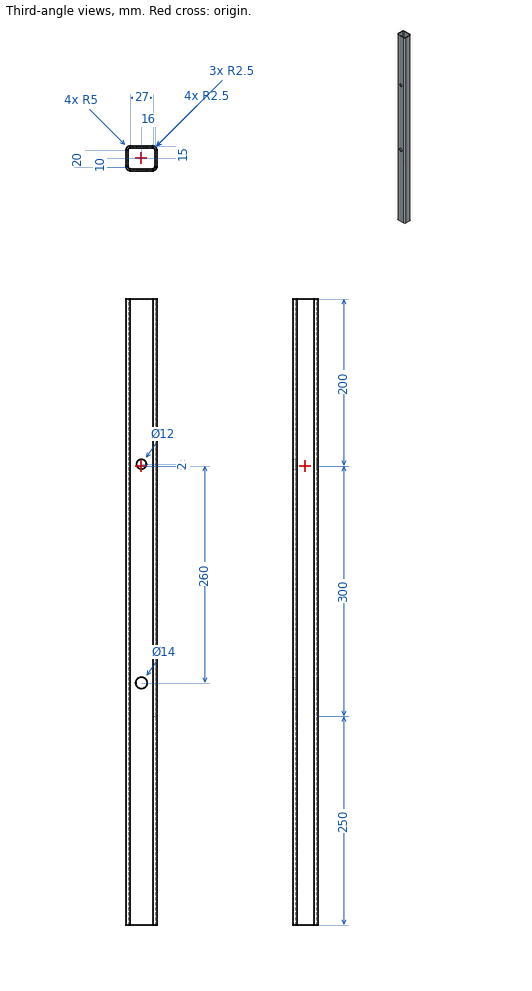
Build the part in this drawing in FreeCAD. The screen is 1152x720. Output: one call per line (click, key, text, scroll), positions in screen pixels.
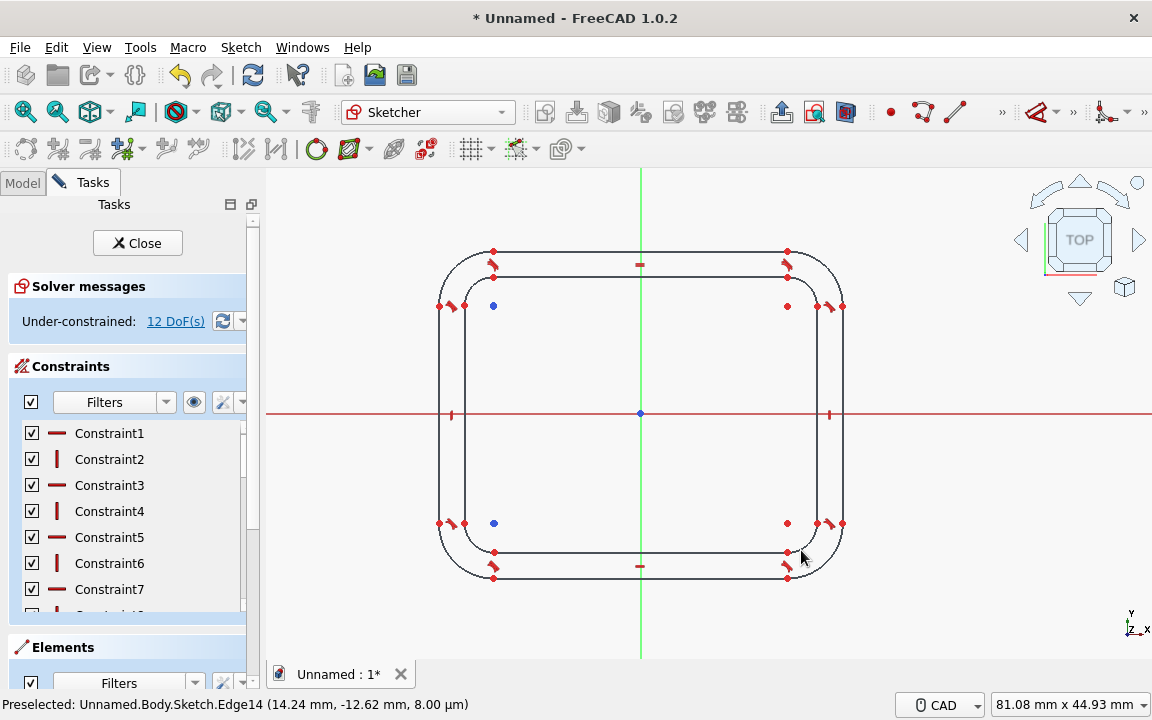
click(445, 549)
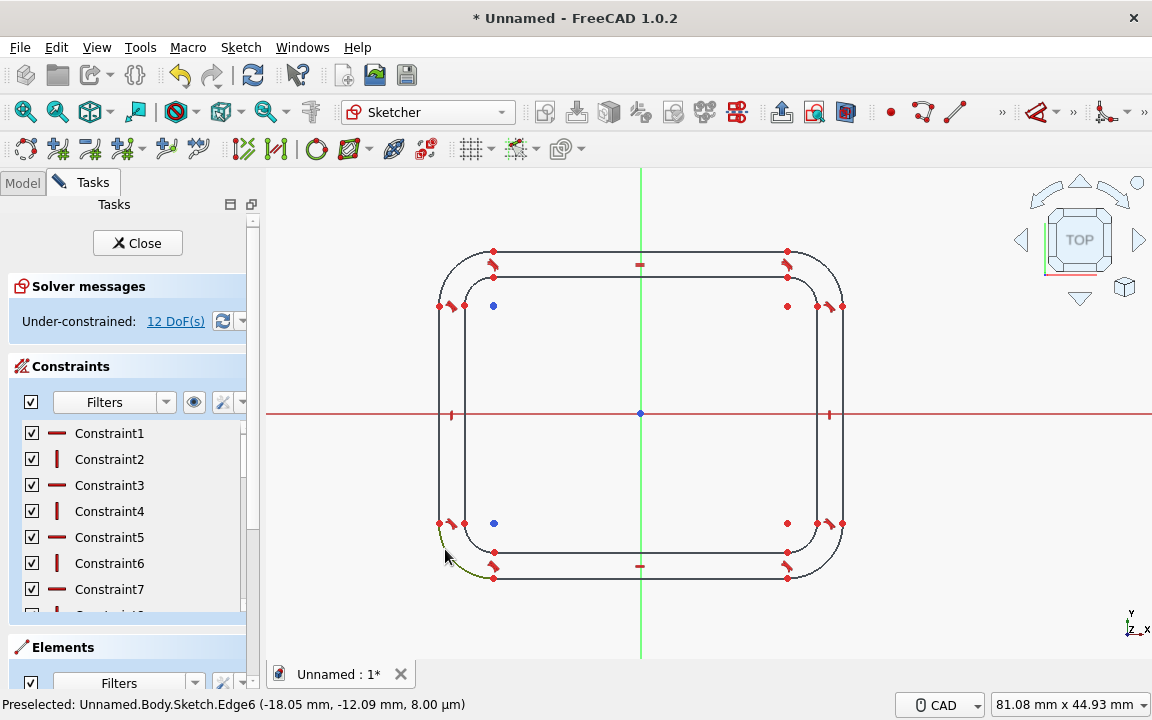
click(468, 537)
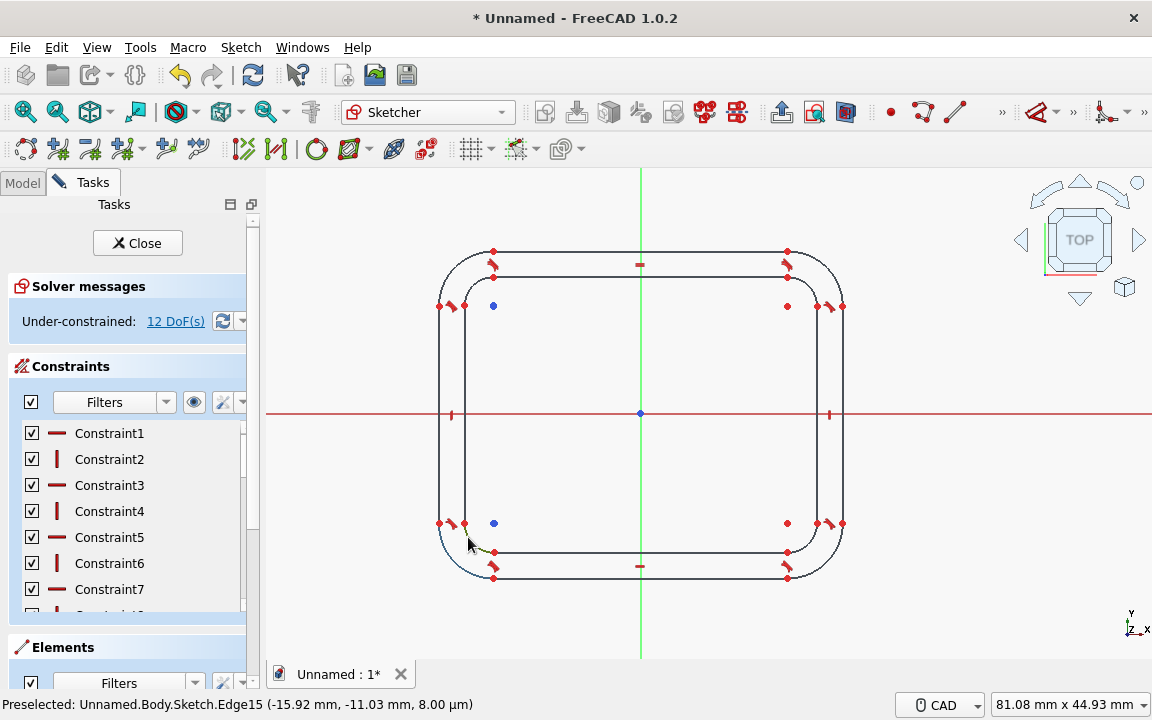
key(c)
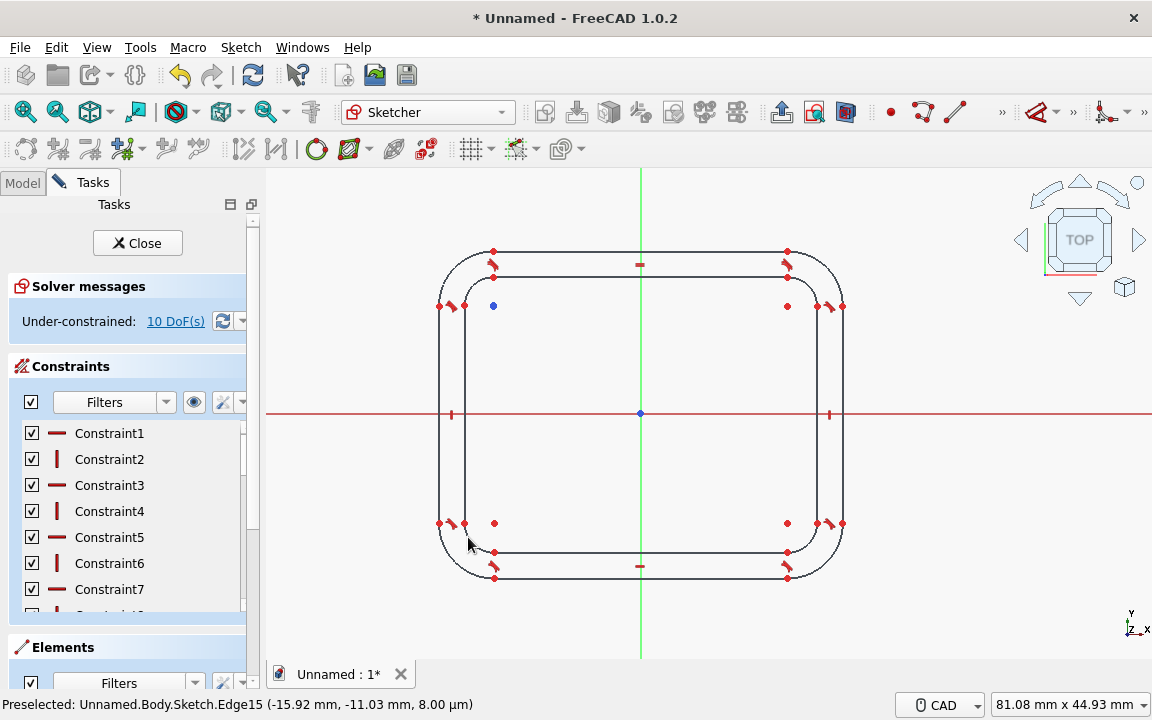
click(469, 257)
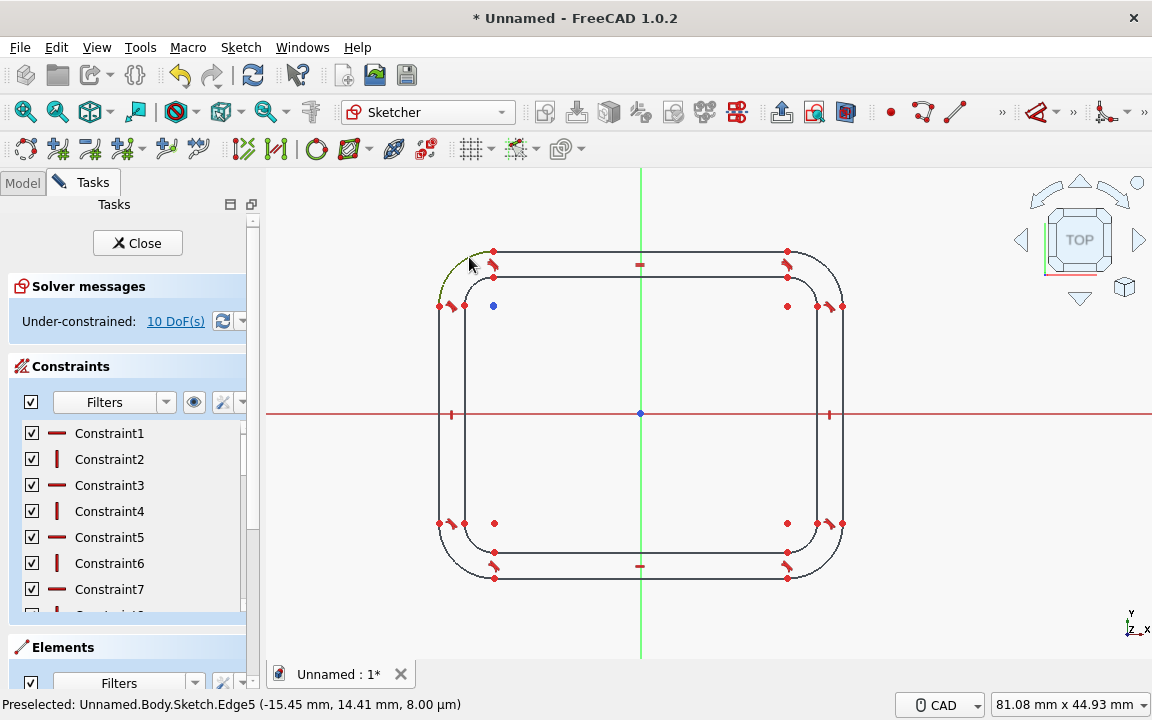
click(445, 548)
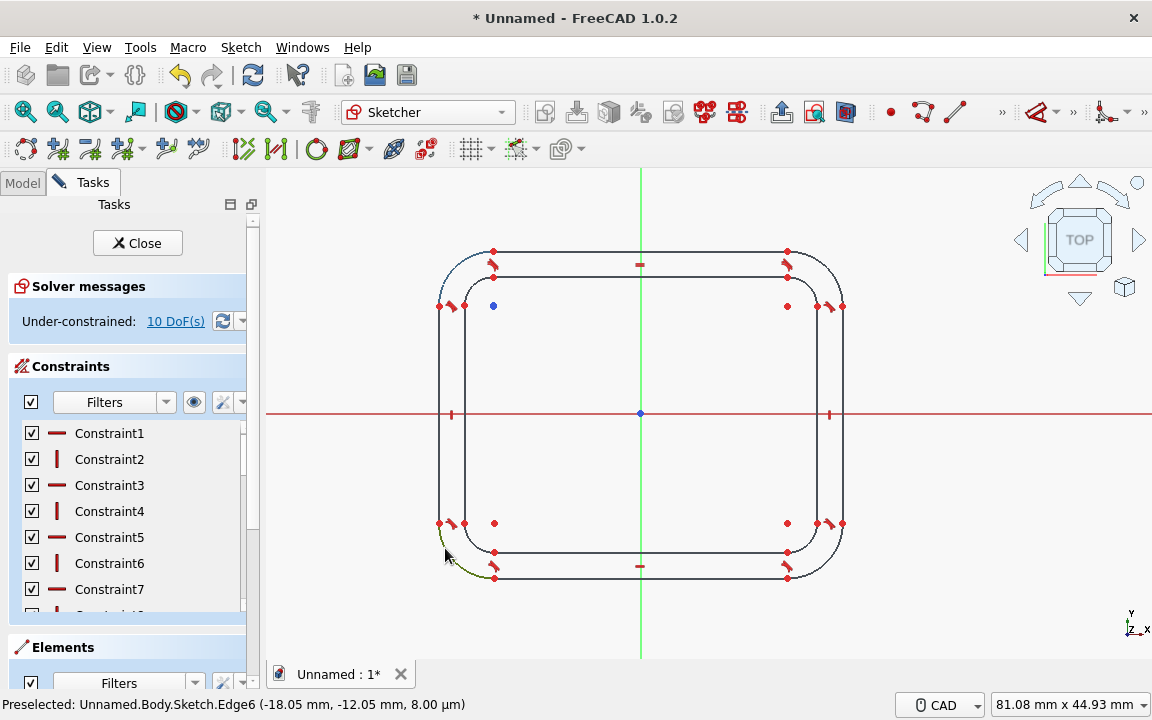
click(812, 573)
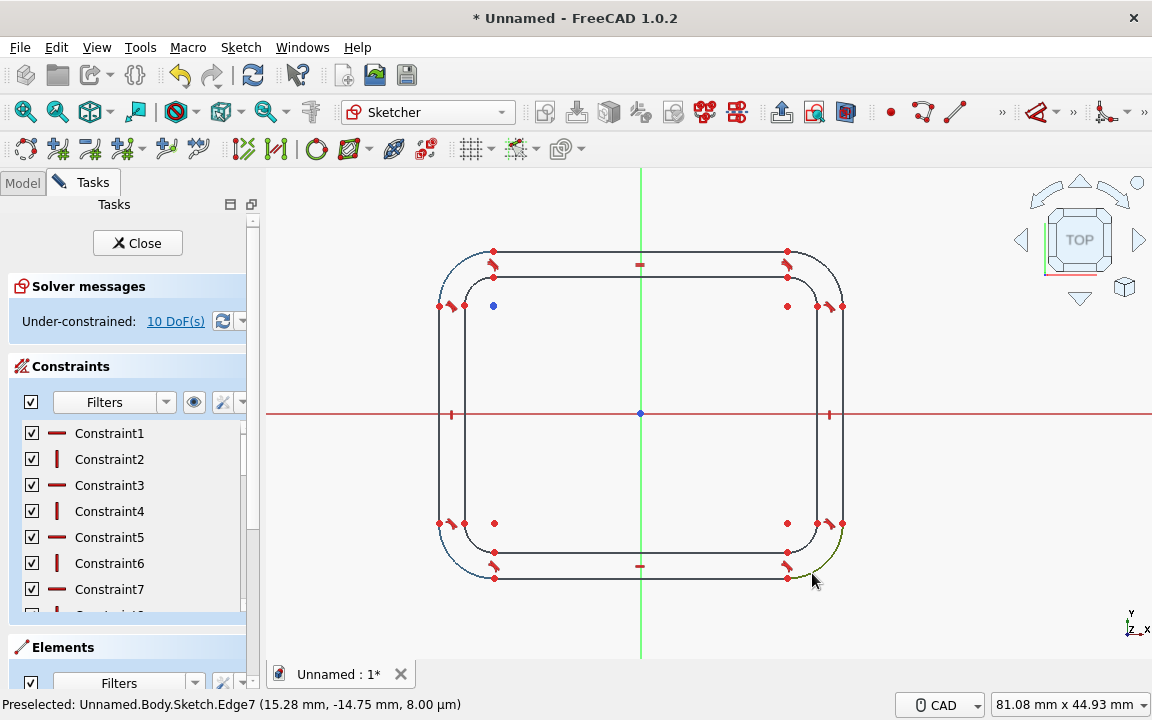
click(837, 281)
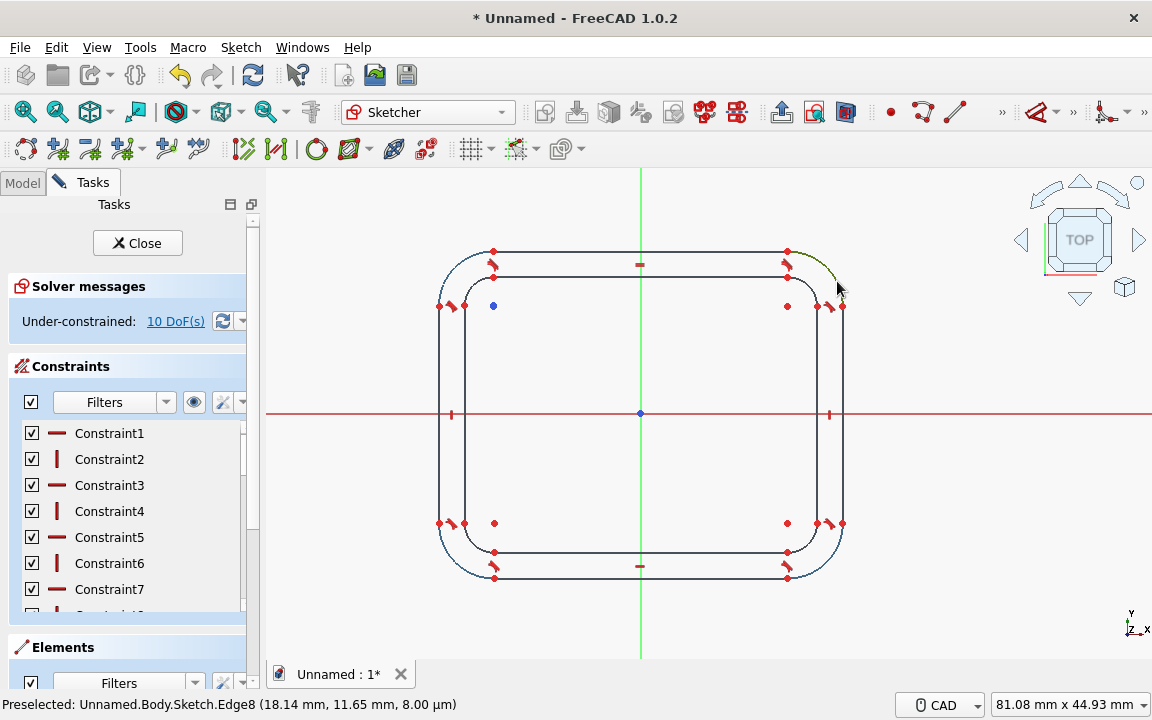
key(e)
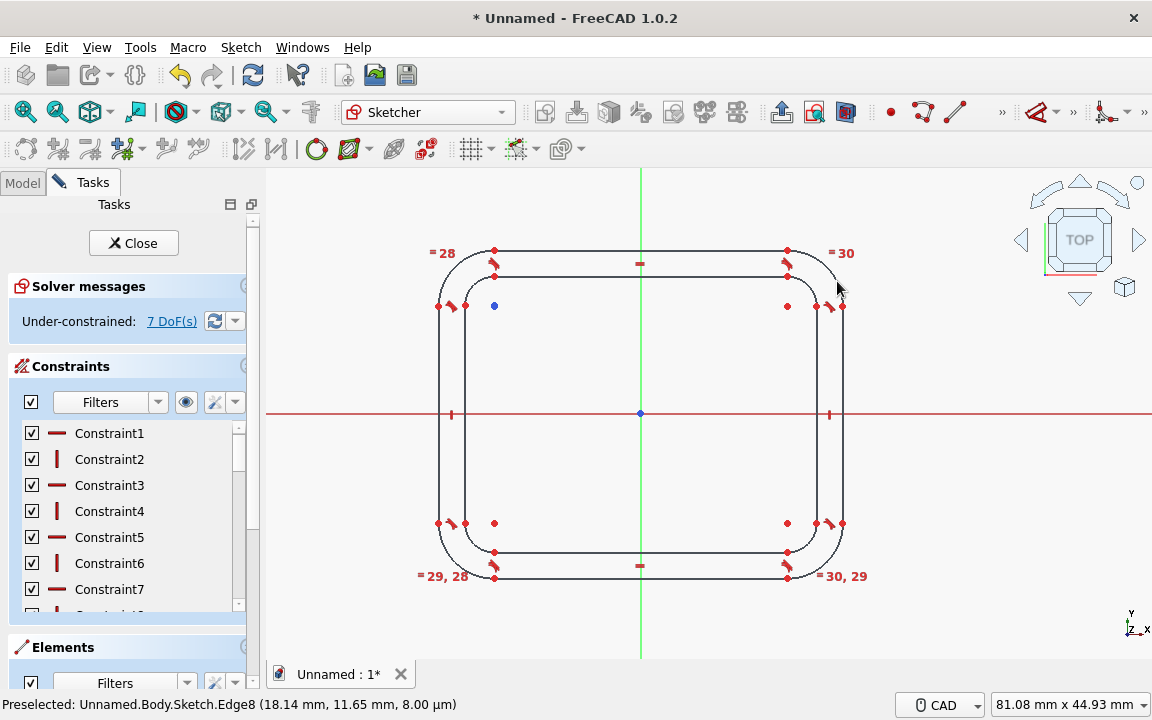
click(814, 293)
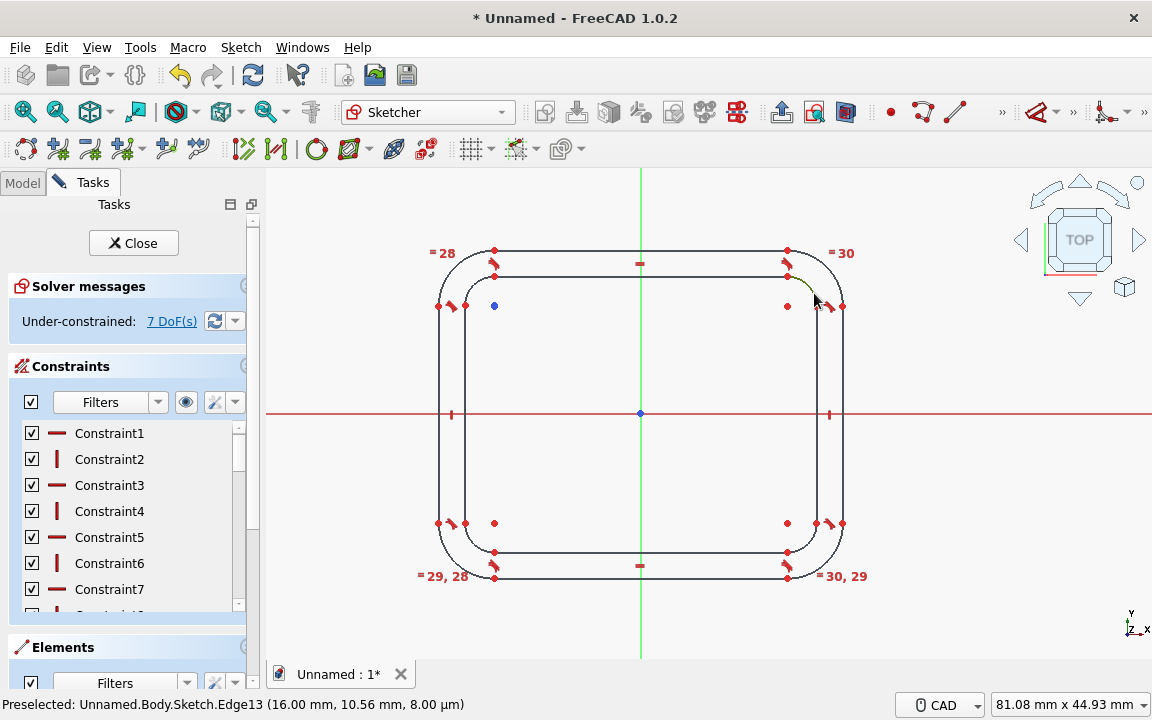
click(481, 280)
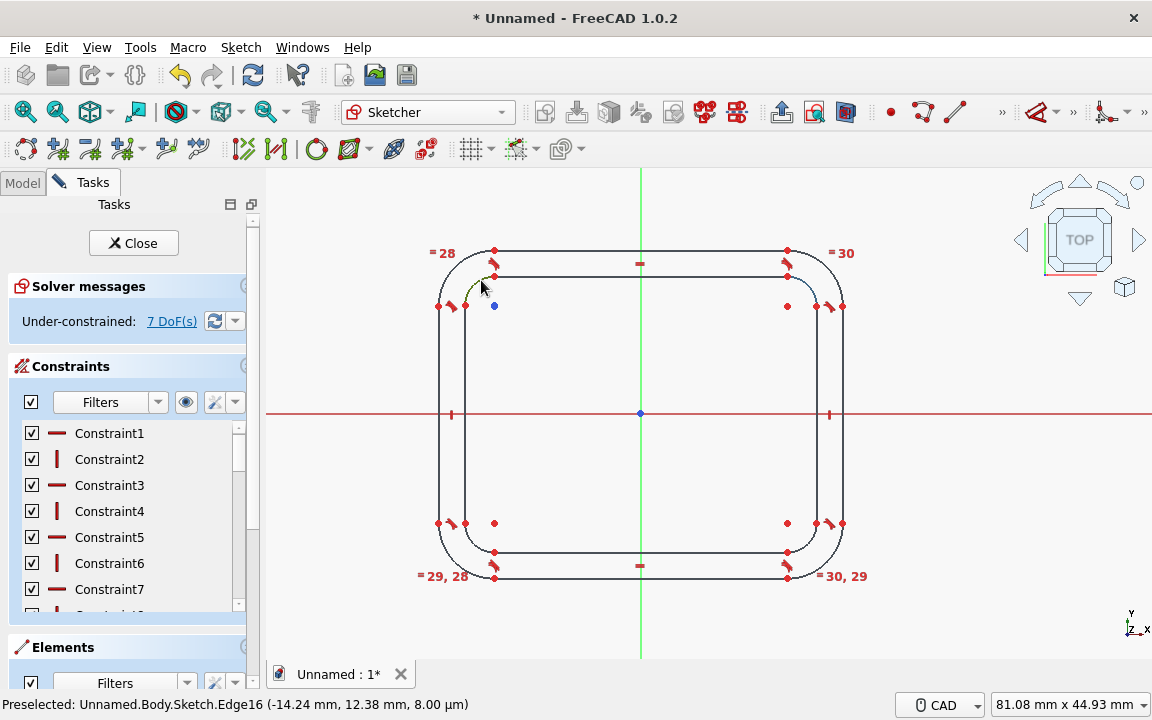
key(e)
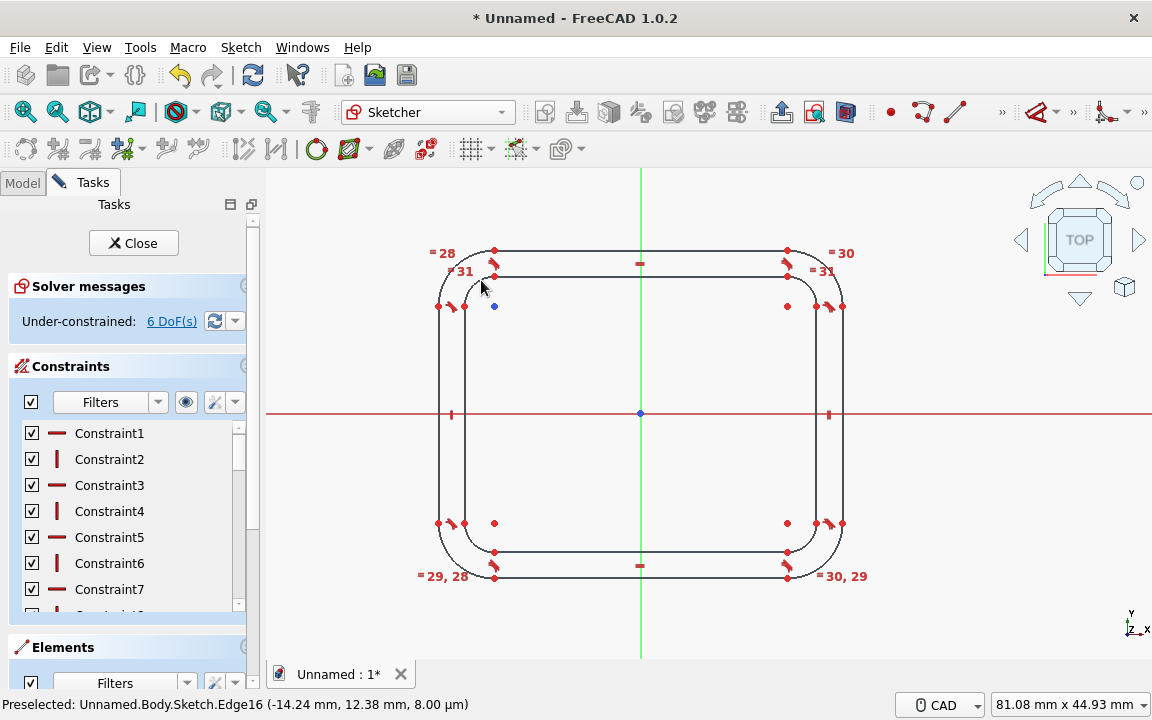
key(d)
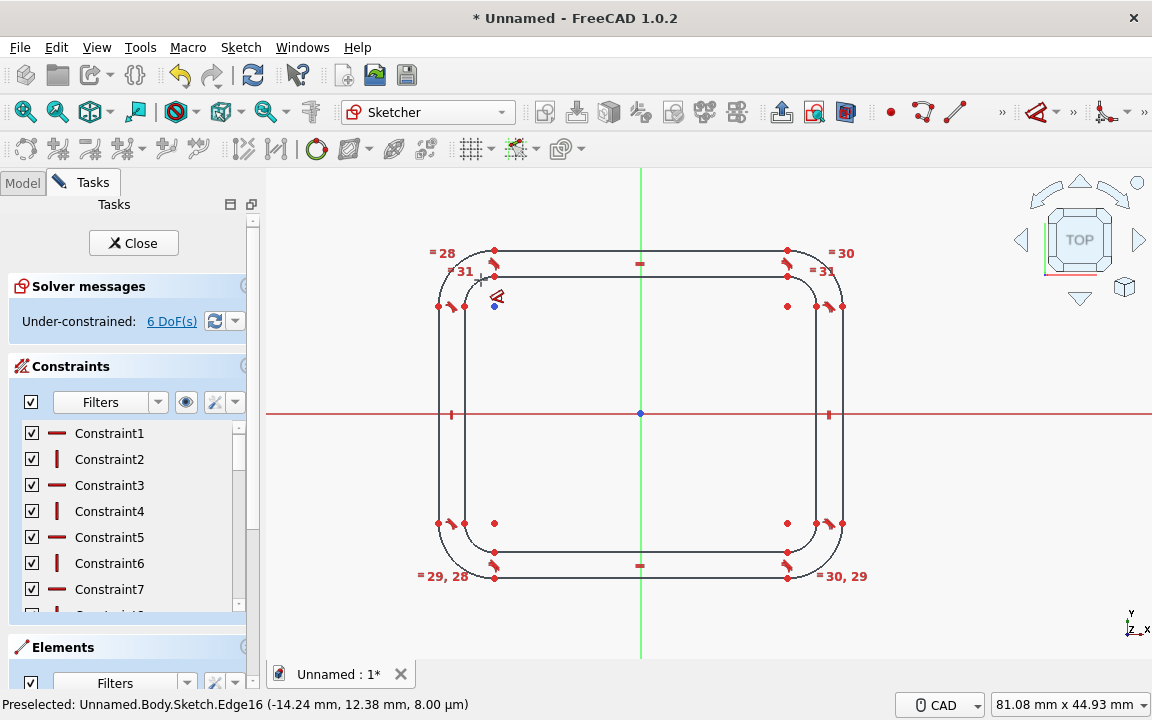
click(469, 257)
click(454, 229)